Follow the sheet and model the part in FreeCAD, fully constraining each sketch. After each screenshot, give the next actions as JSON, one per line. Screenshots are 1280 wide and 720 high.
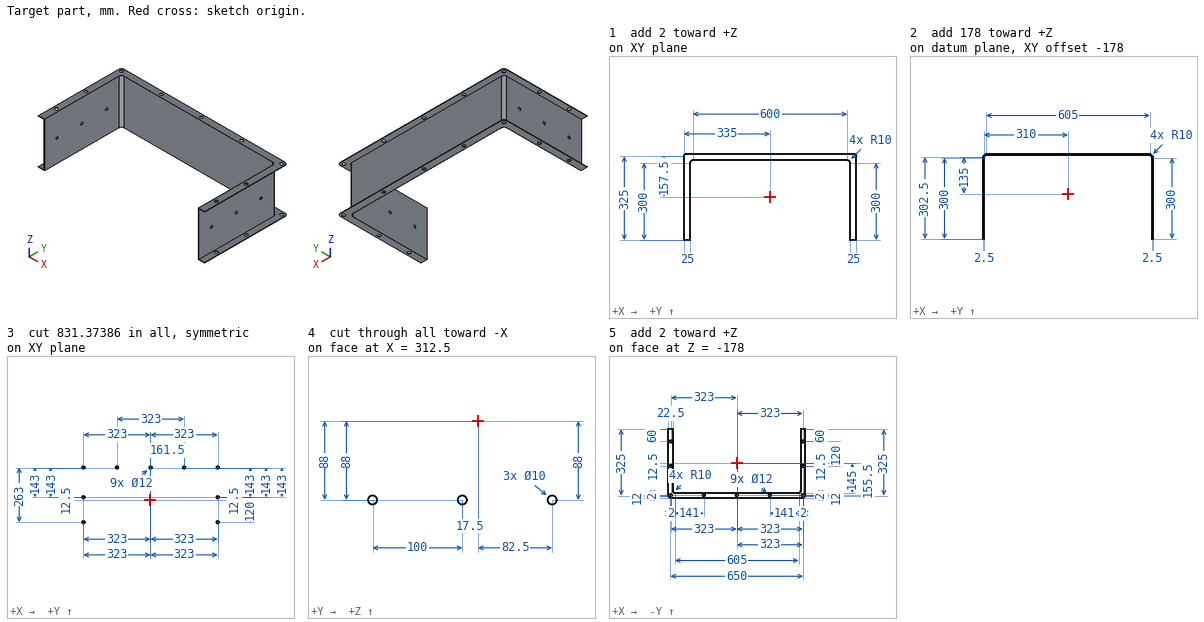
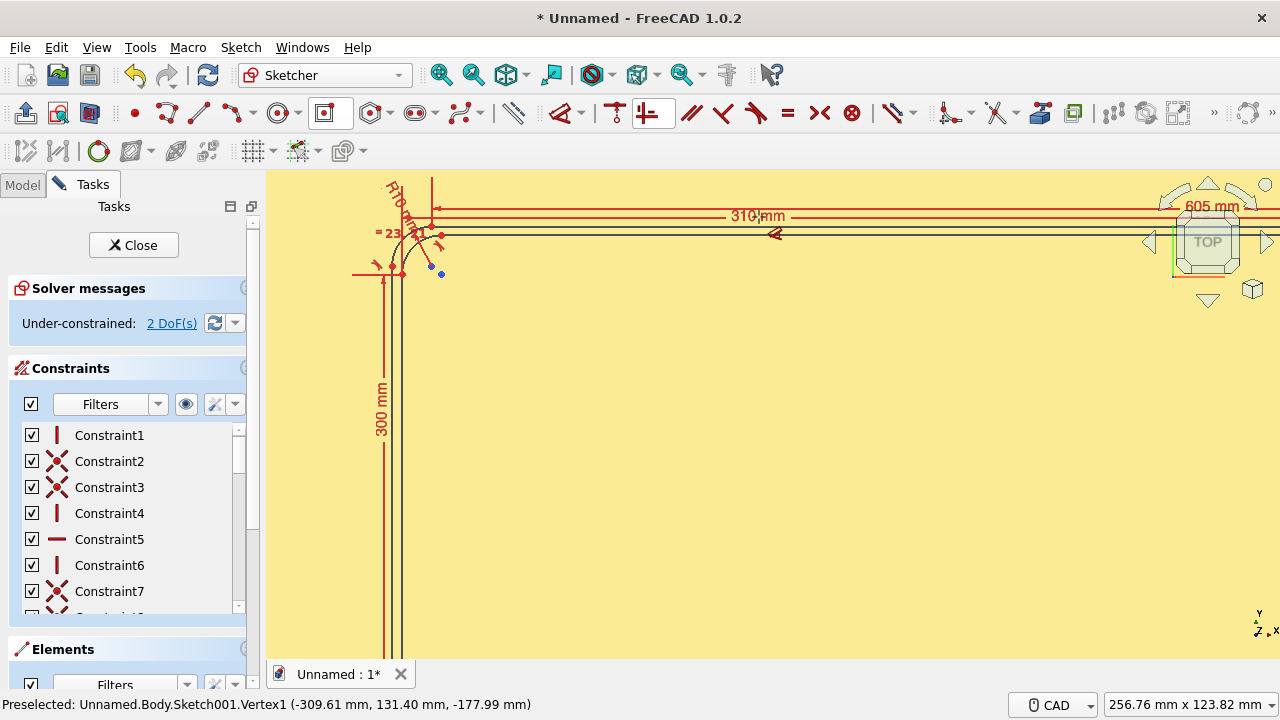
{"action": "left_click", "coordinate": [392, 266]}
{"action": "left_click", "coordinate": [358, 449]}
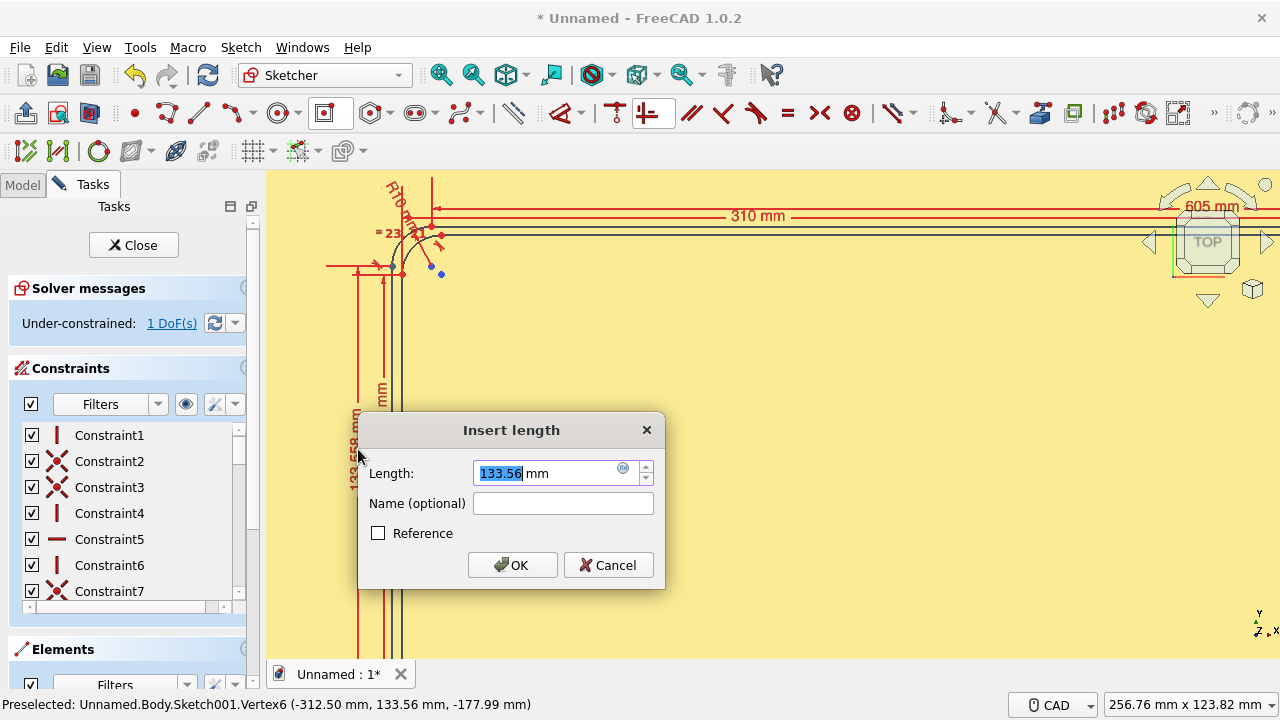
{"action": "type", "text": "135"}
{"action": "key", "text": "Return"}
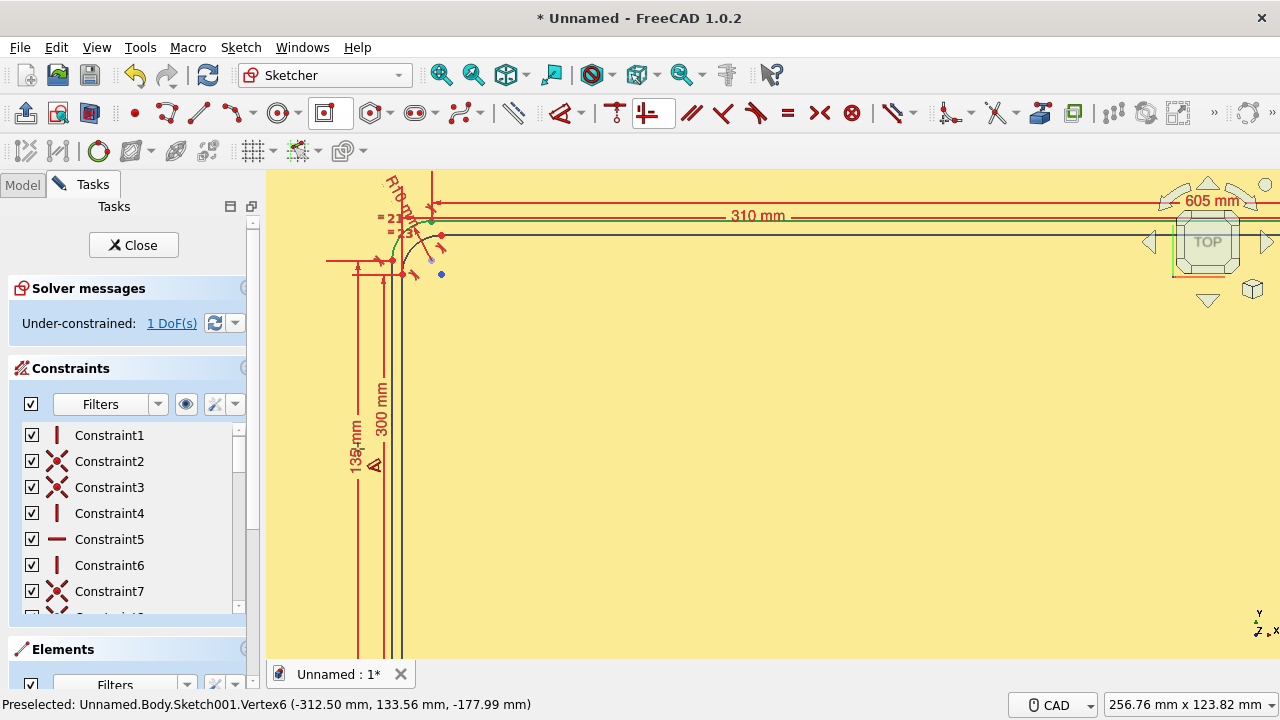
{"action": "scroll", "coordinate": [392, 620], "scroll_direction": "up", "scroll_amount": 2}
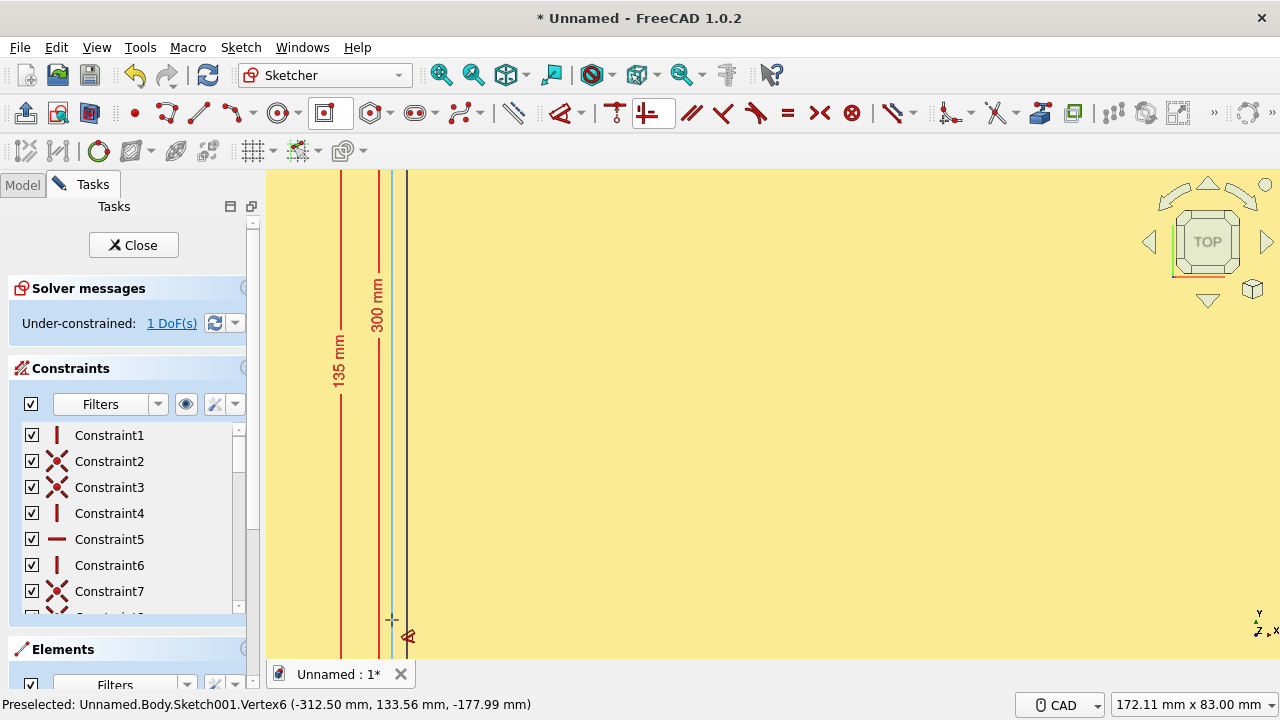
{"action": "left_click", "coordinate": [392, 620]}
{"action": "left_click", "coordinate": [358, 414]}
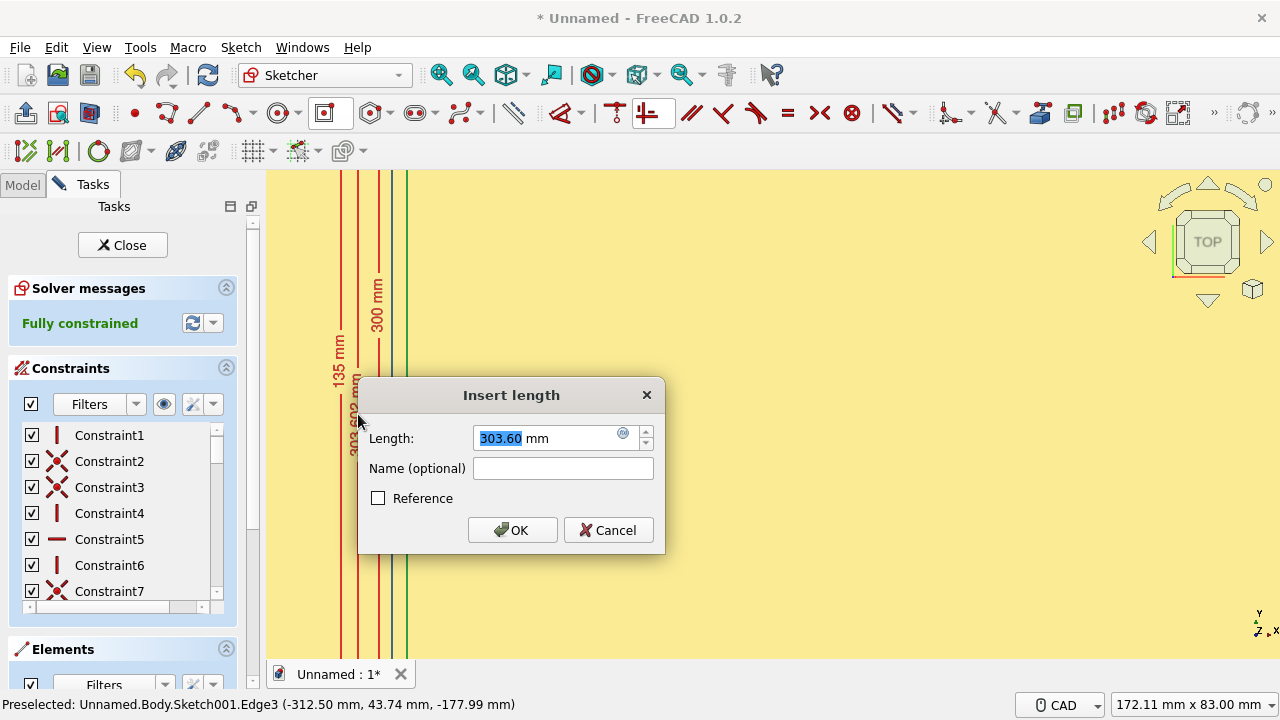
{"action": "type", "text": "302.5"}
{"action": "key", "text": "Return"}
{"action": "key", "text": "Escape"}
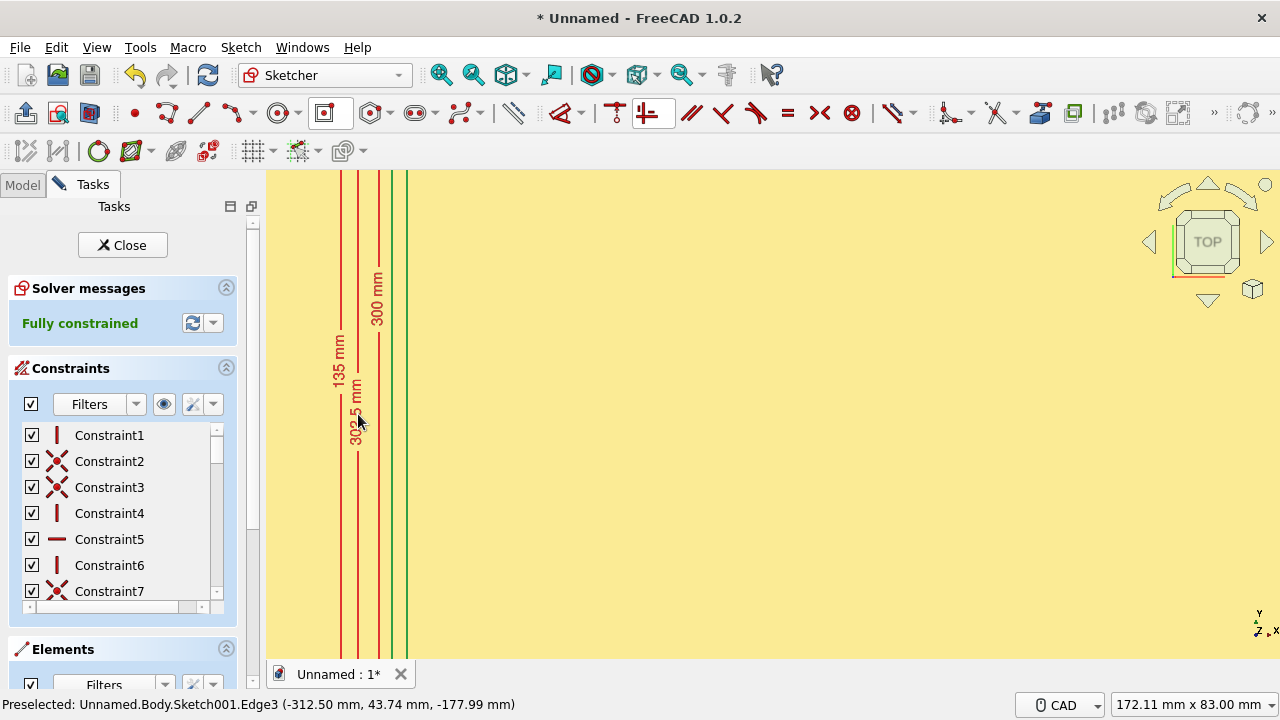
{"action": "left_click", "coordinate": [123, 245]}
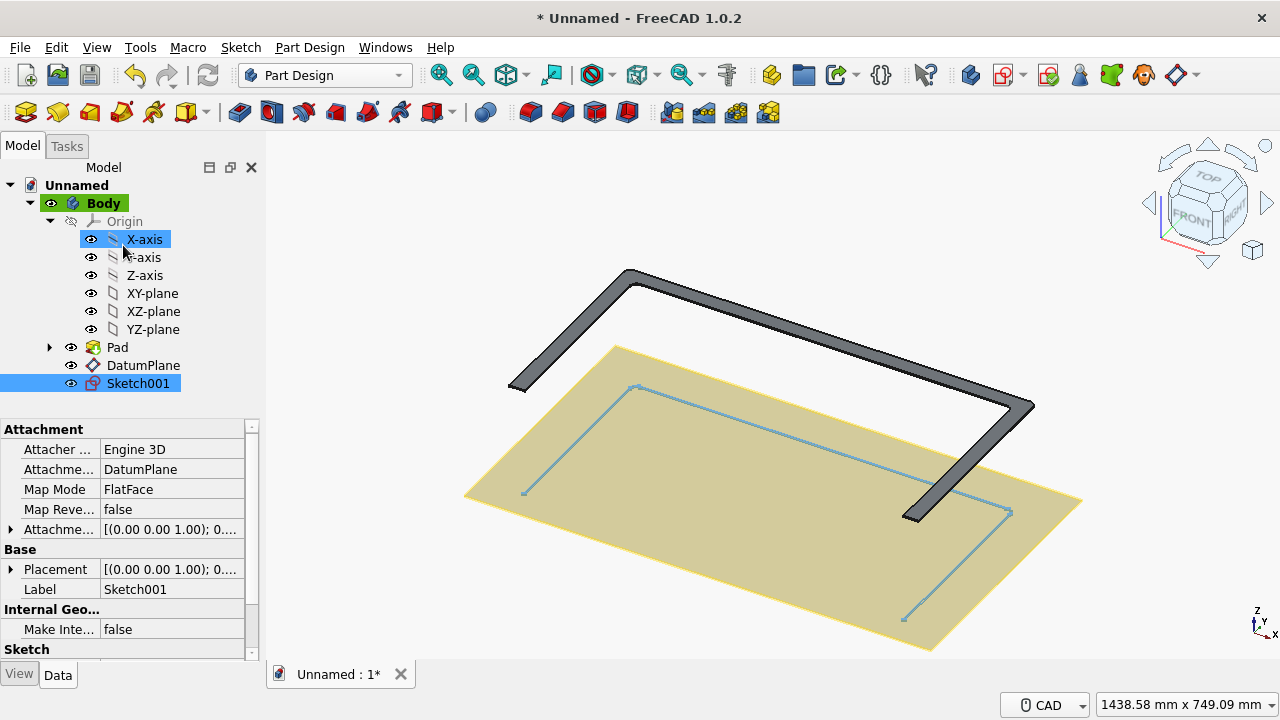
{"action": "left_click", "coordinate": [26, 112]}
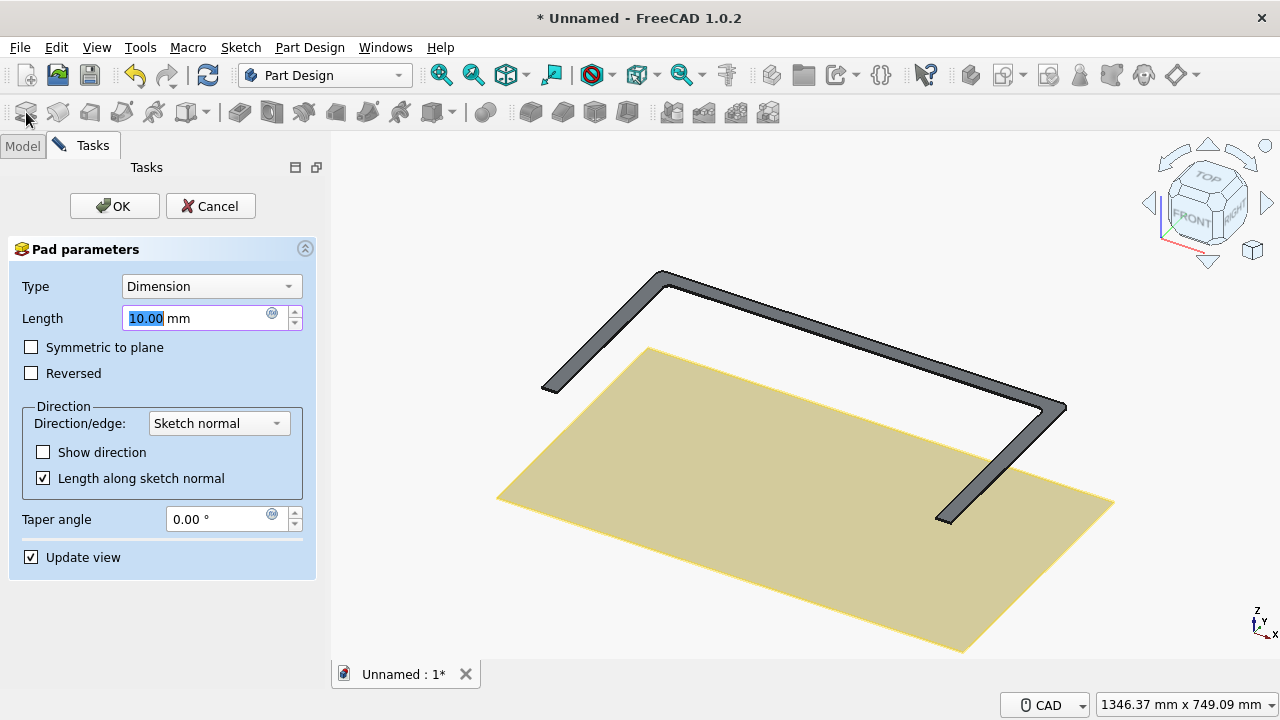
{"action": "type", "text": "178"}
{"action": "key", "text": "Tab"}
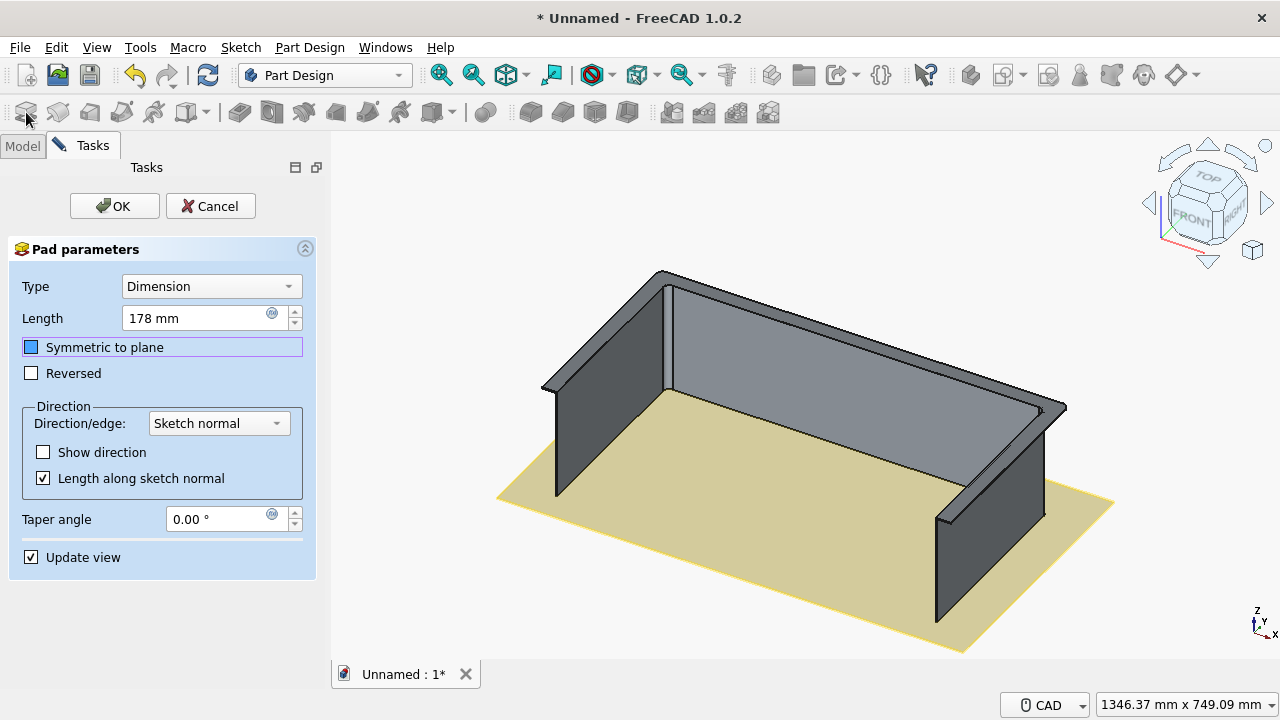
{"action": "left_click", "coordinate": [115, 206]}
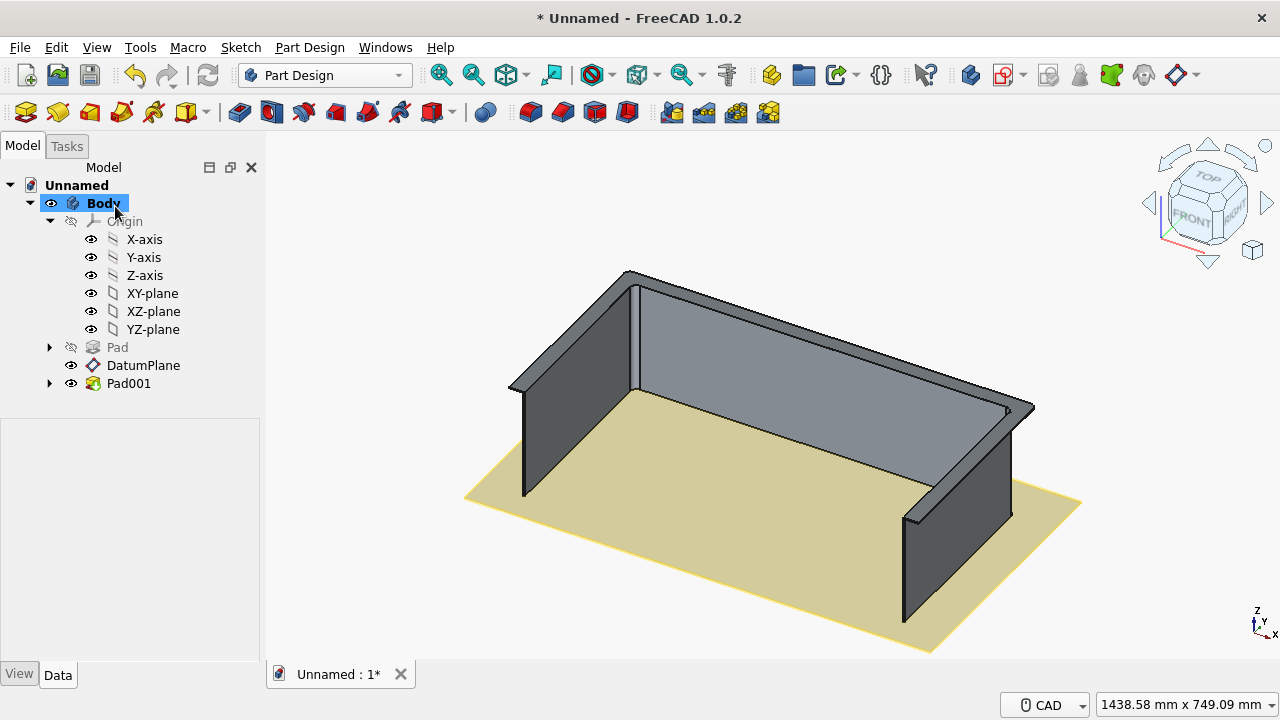
{"action": "left_click", "coordinate": [116, 365]}
{"action": "key", "text": "space"}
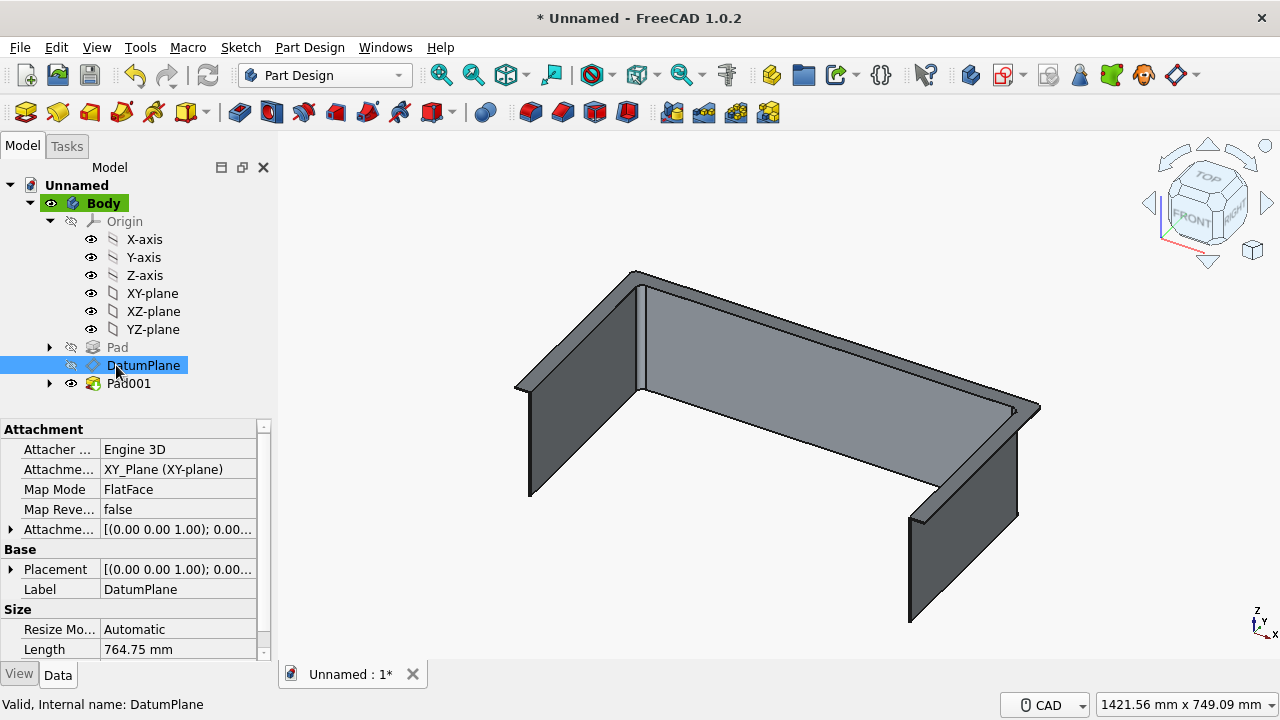
{"action": "key", "text": "5"}